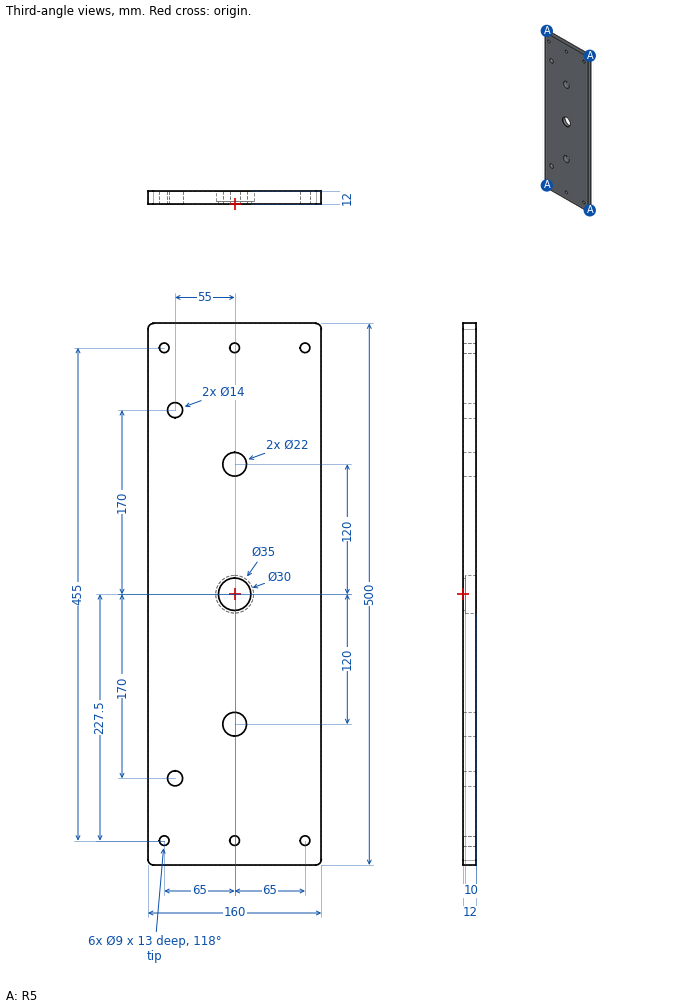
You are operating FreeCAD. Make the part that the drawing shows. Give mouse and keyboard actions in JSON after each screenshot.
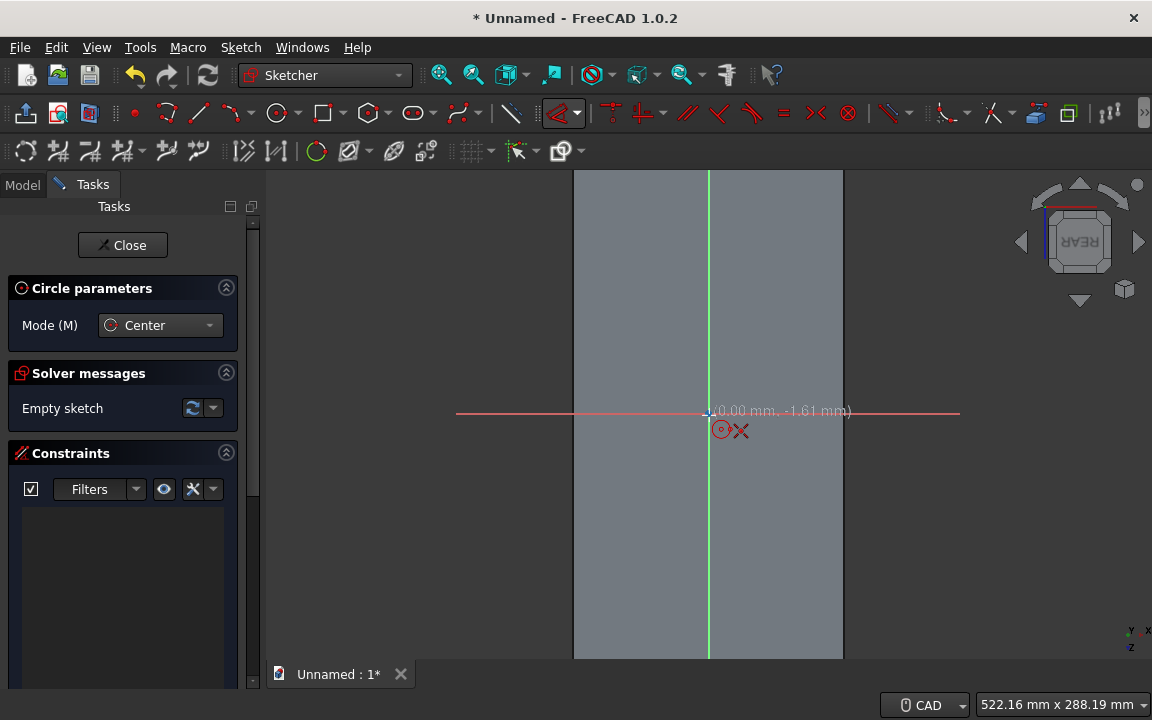
{"action": "left_click", "coordinate": [709, 414]}
{"action": "left_click", "coordinate": [727, 396]}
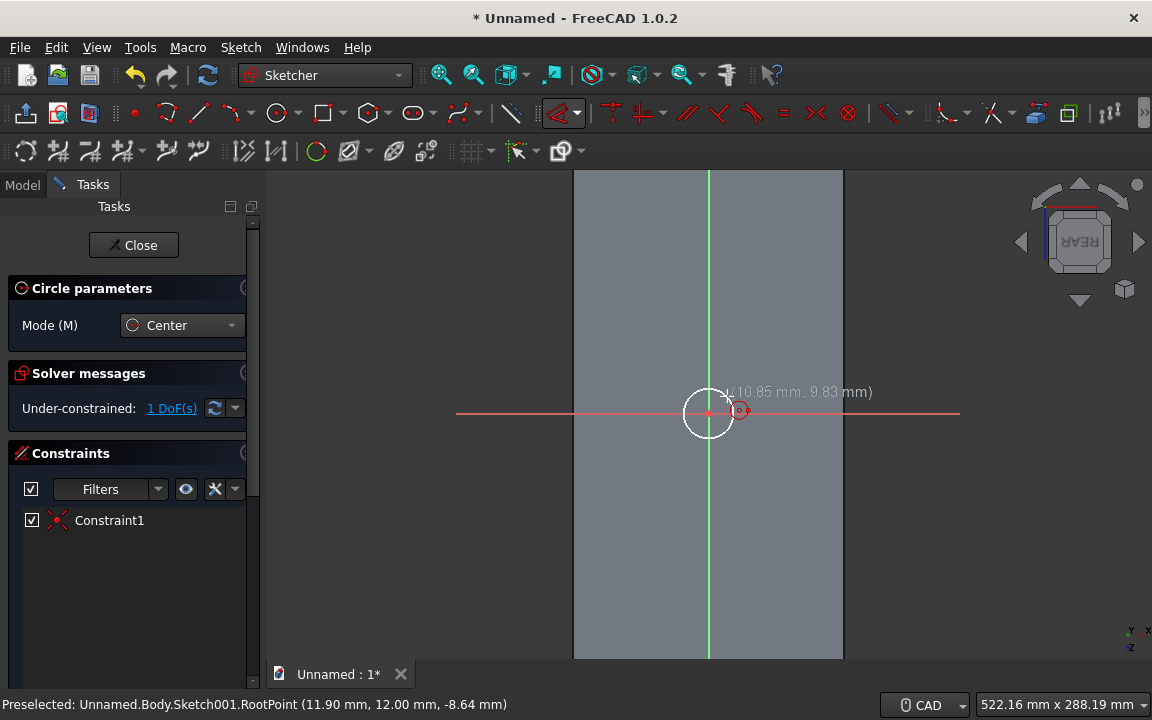
{"action": "left_click", "coordinate": [709, 617]}
{"action": "left_click", "coordinate": [726, 611]}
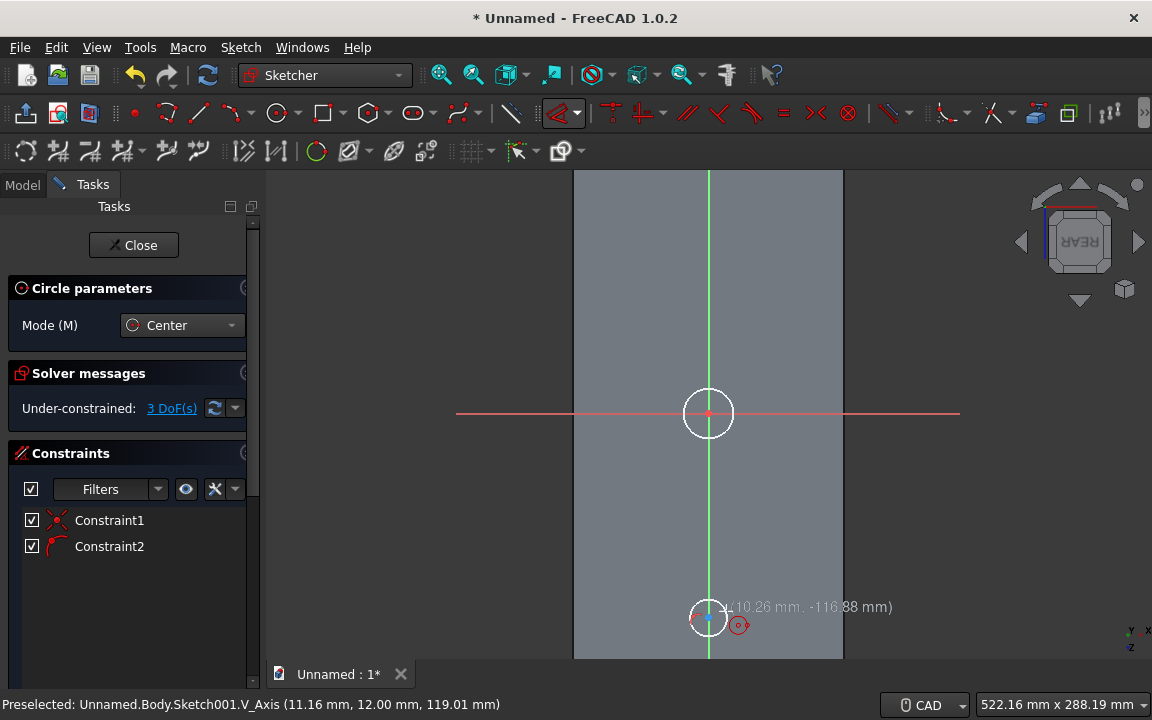
{"action": "left_click", "coordinate": [709, 210]}
{"action": "left_click", "coordinate": [726, 204]}
{"action": "key", "text": "Escape"}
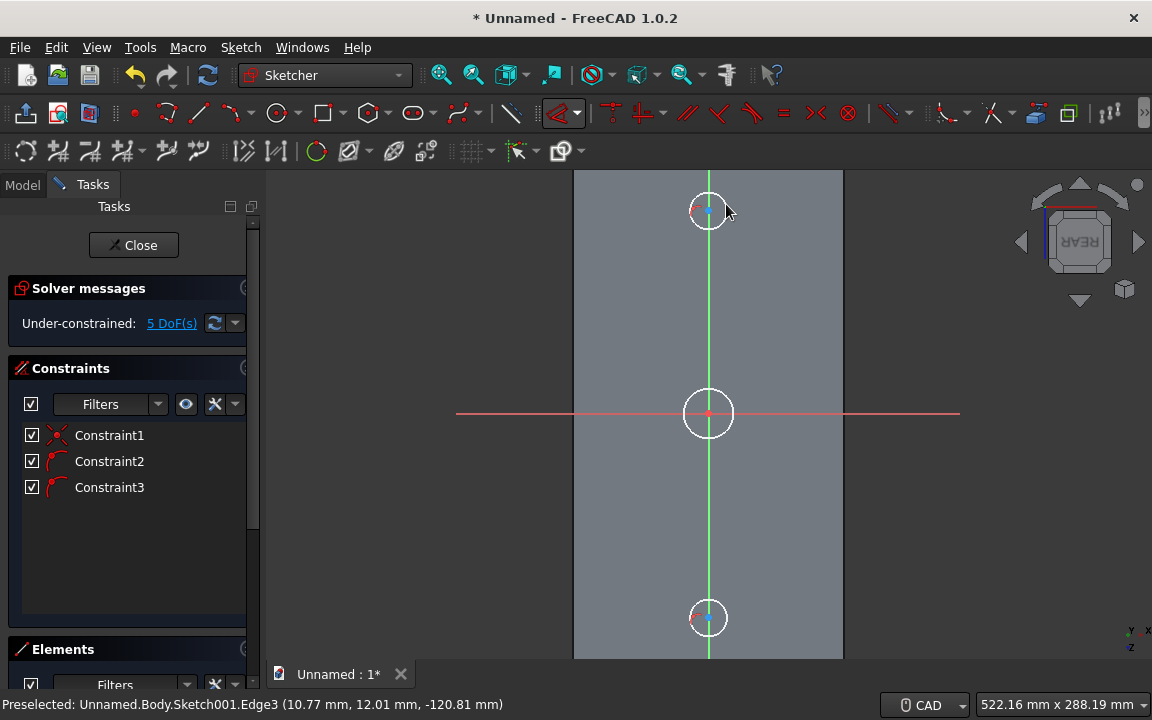
{"action": "left_click", "coordinate": [722, 605]}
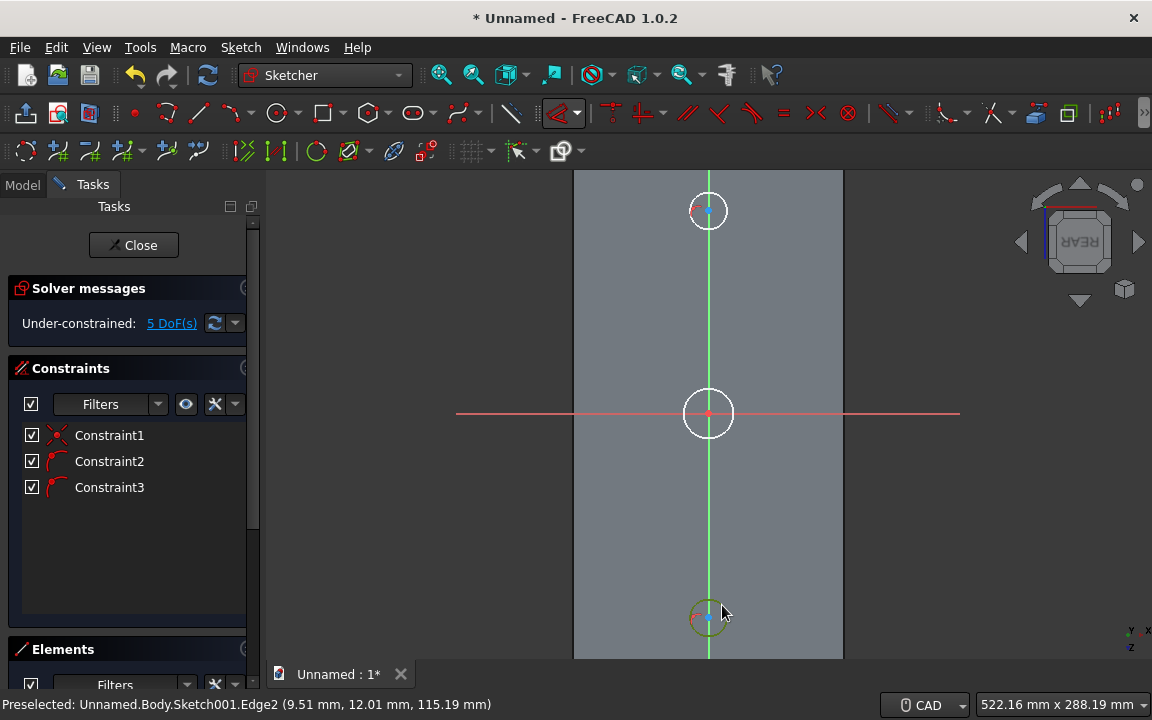
{"action": "left_click", "coordinate": [696, 198]}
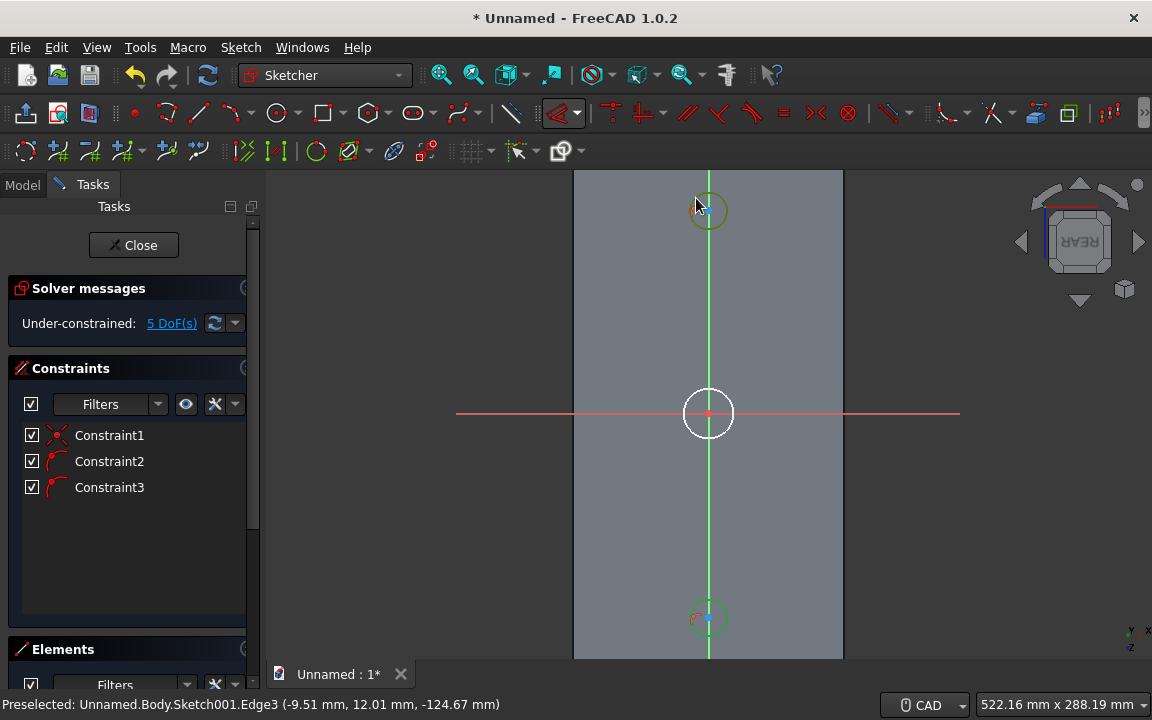
{"action": "left_click", "coordinate": [784, 114]}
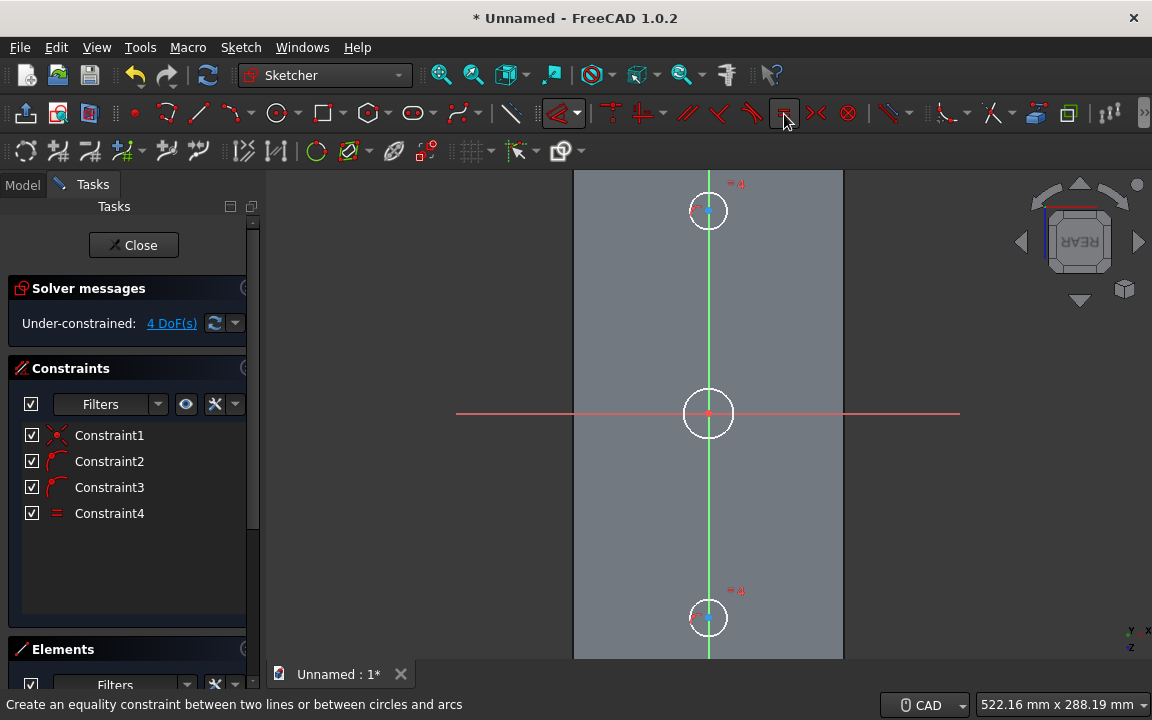
{"action": "left_click", "coordinate": [726, 396]}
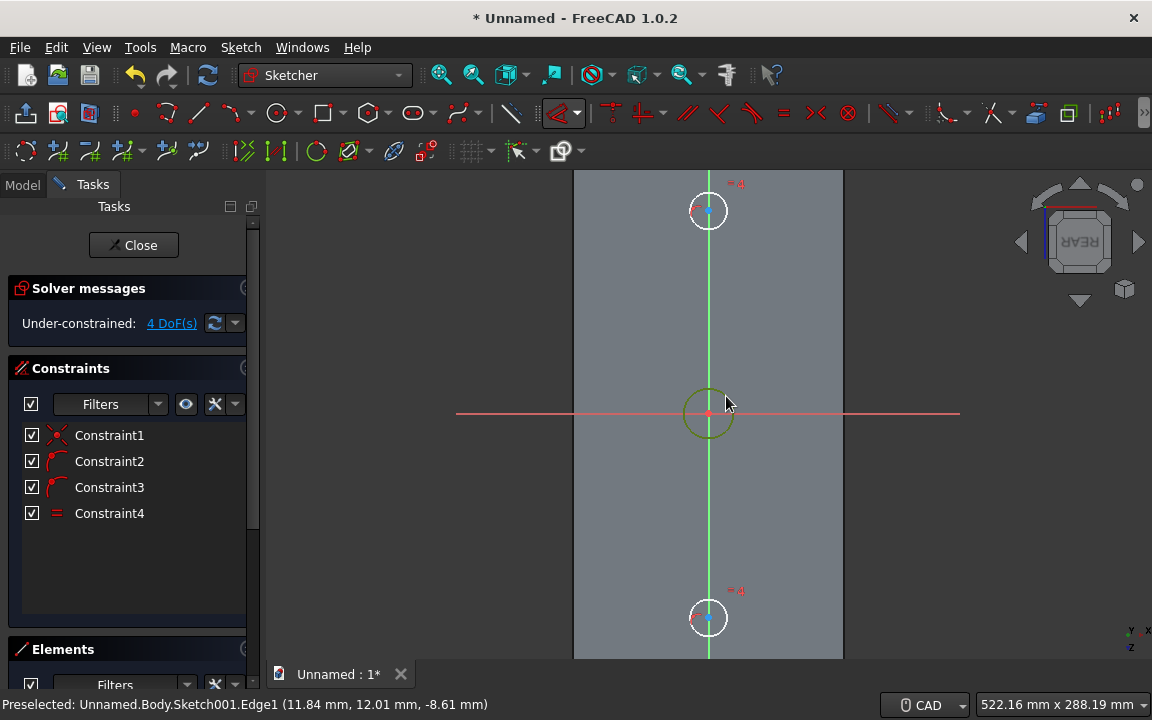
{"action": "left_click", "coordinate": [580, 114]}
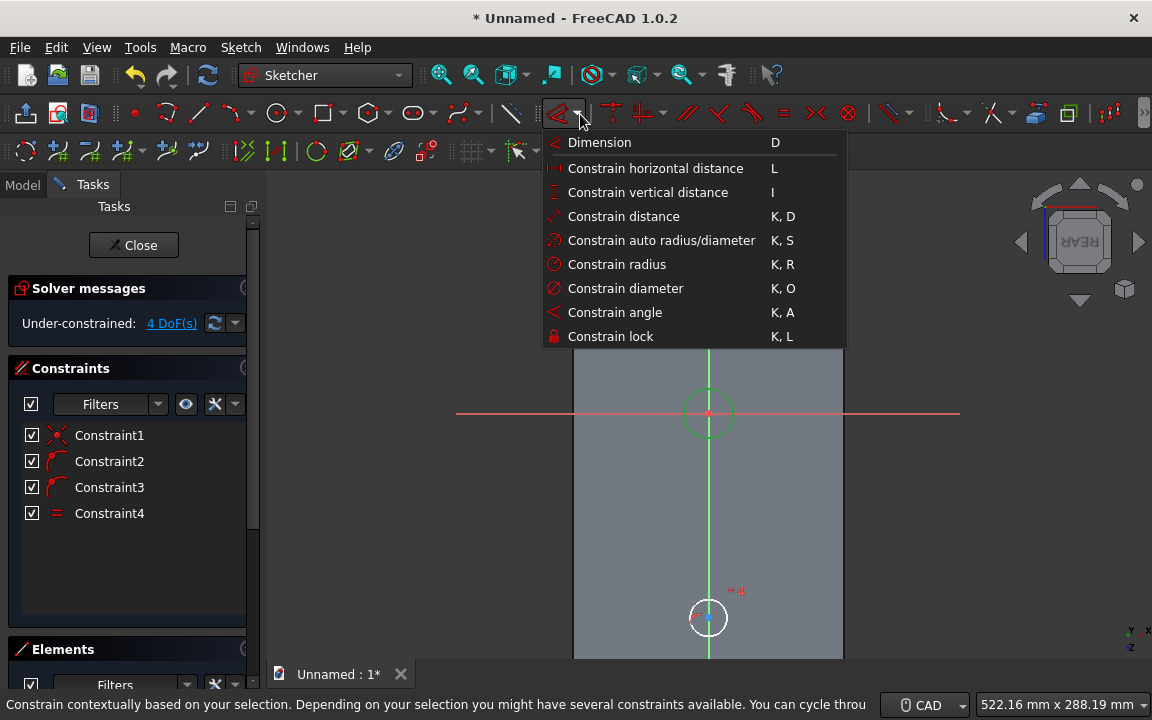
{"action": "left_click", "coordinate": [695, 288]}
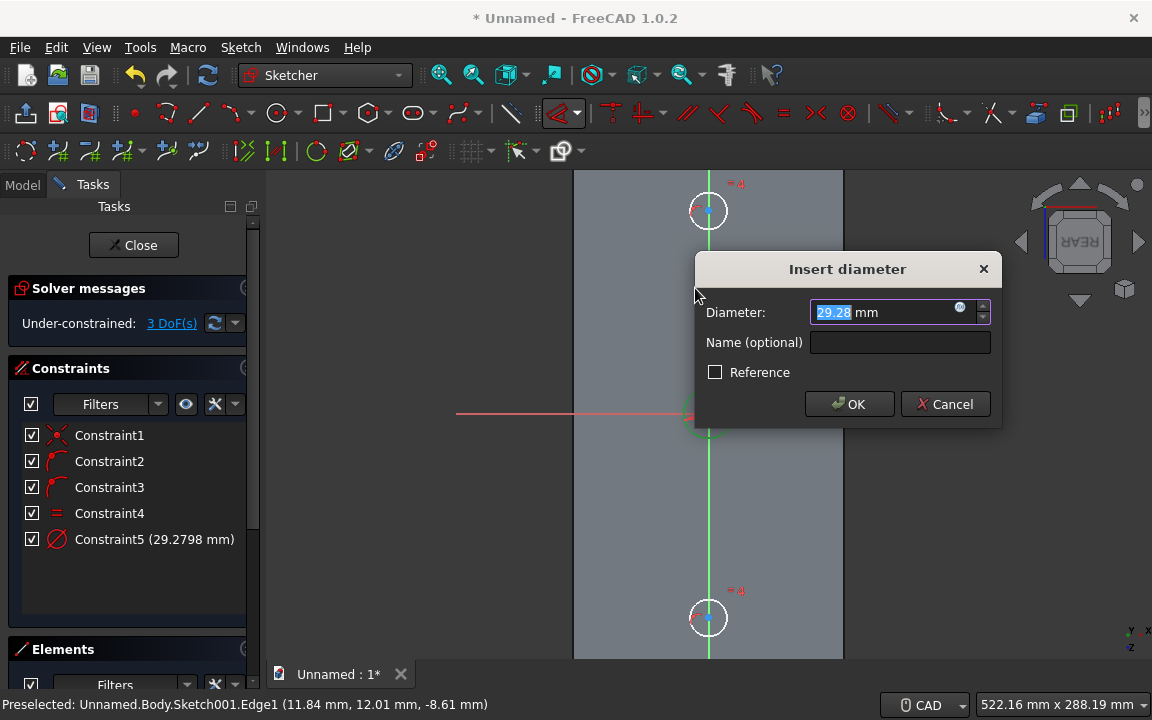
{"action": "type", "text": "30"}
{"action": "key", "text": "Return"}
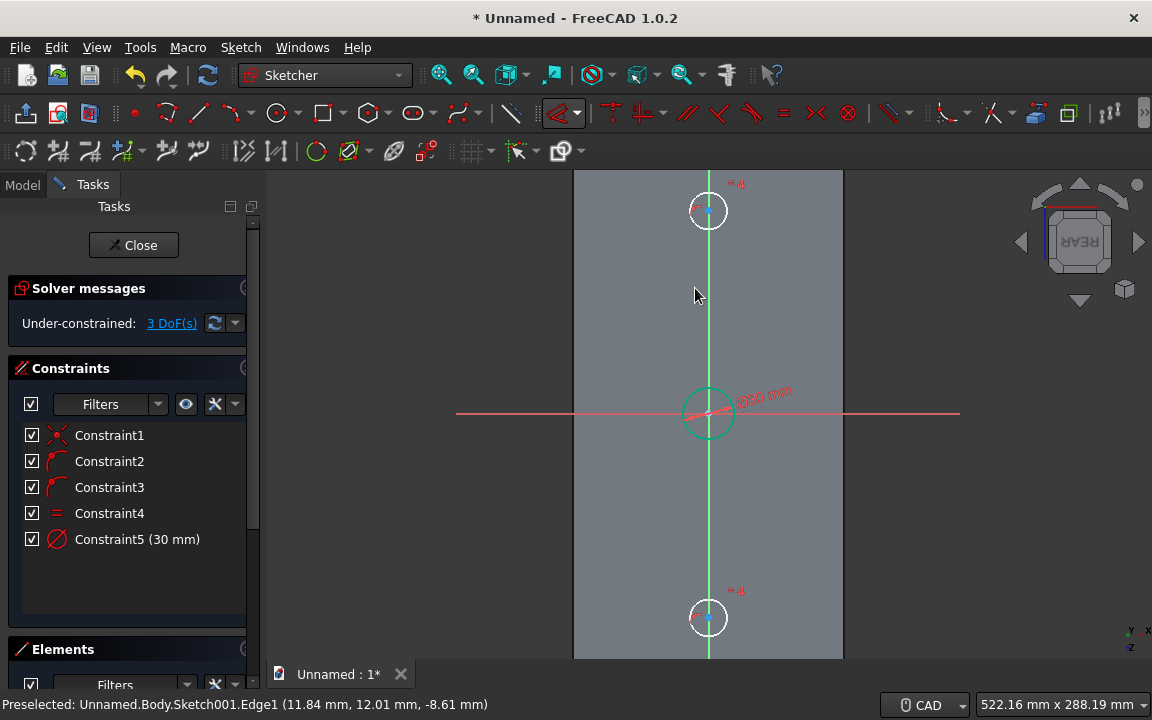
{"action": "left_click", "coordinate": [722, 605]}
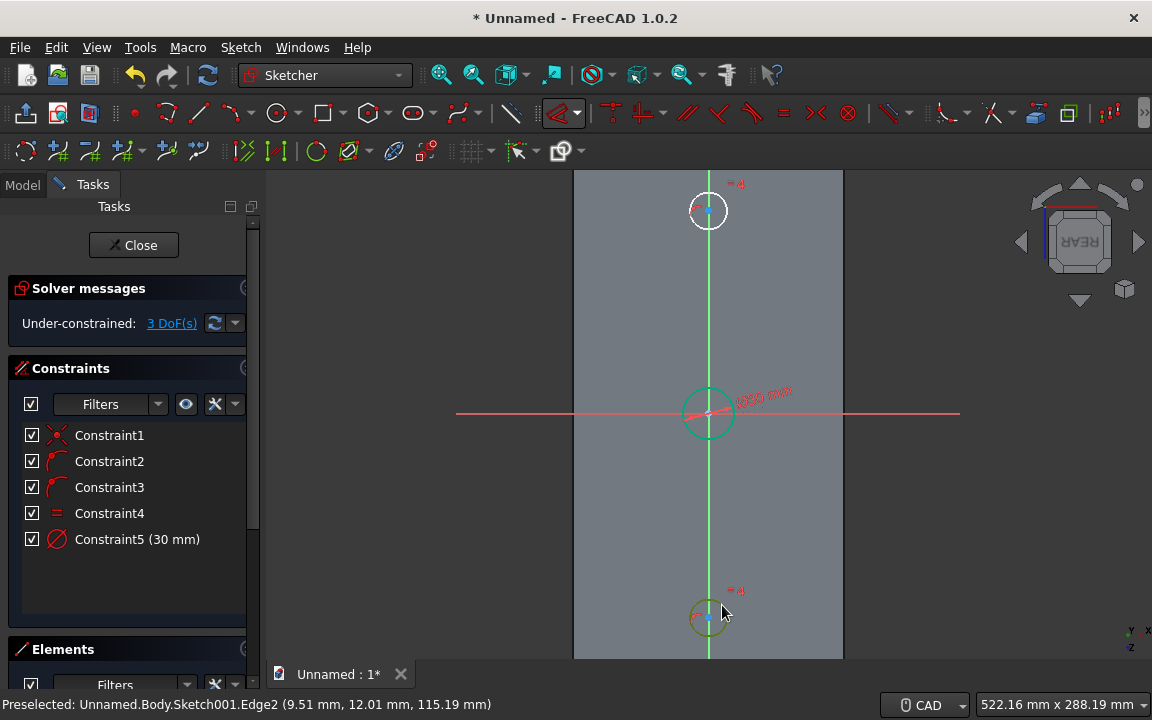
{"action": "key", "text": "k o"}